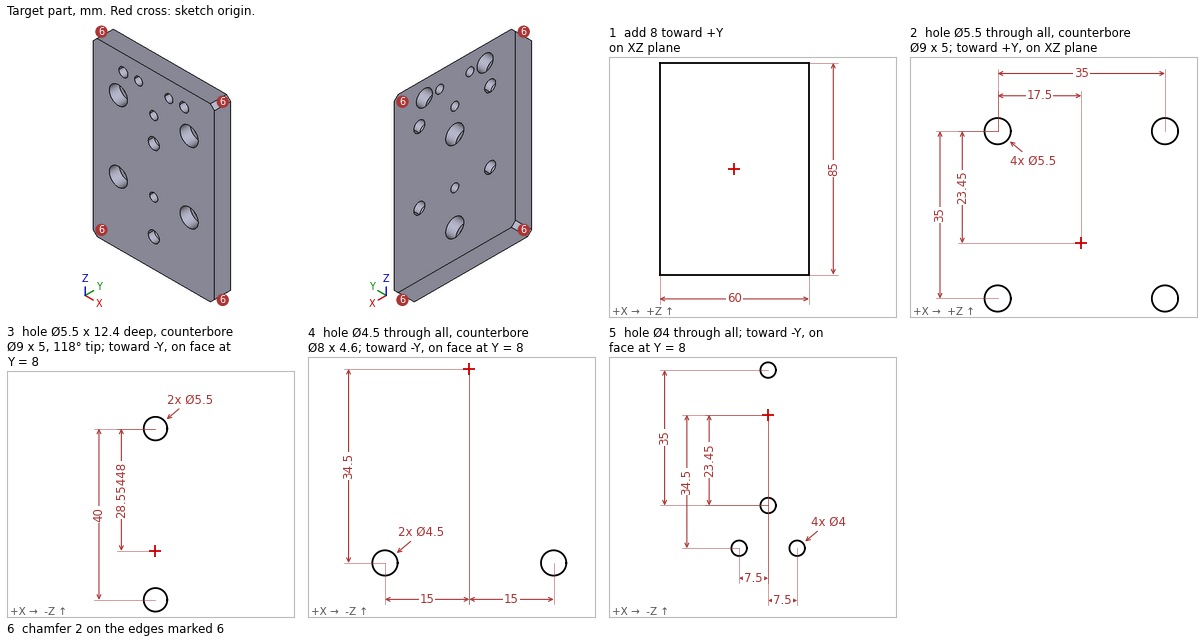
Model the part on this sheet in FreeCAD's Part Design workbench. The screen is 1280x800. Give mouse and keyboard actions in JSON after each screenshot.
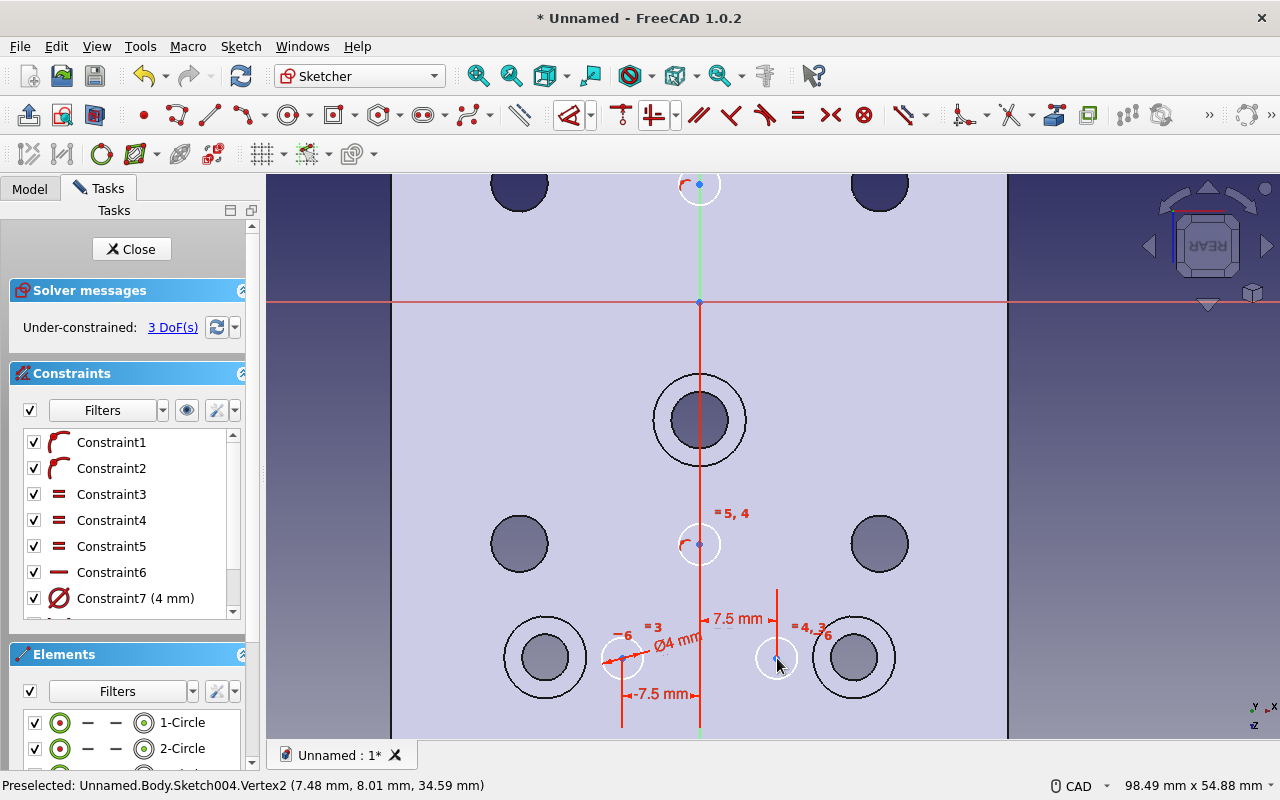
{"action": "left_click", "coordinate": [700, 545]}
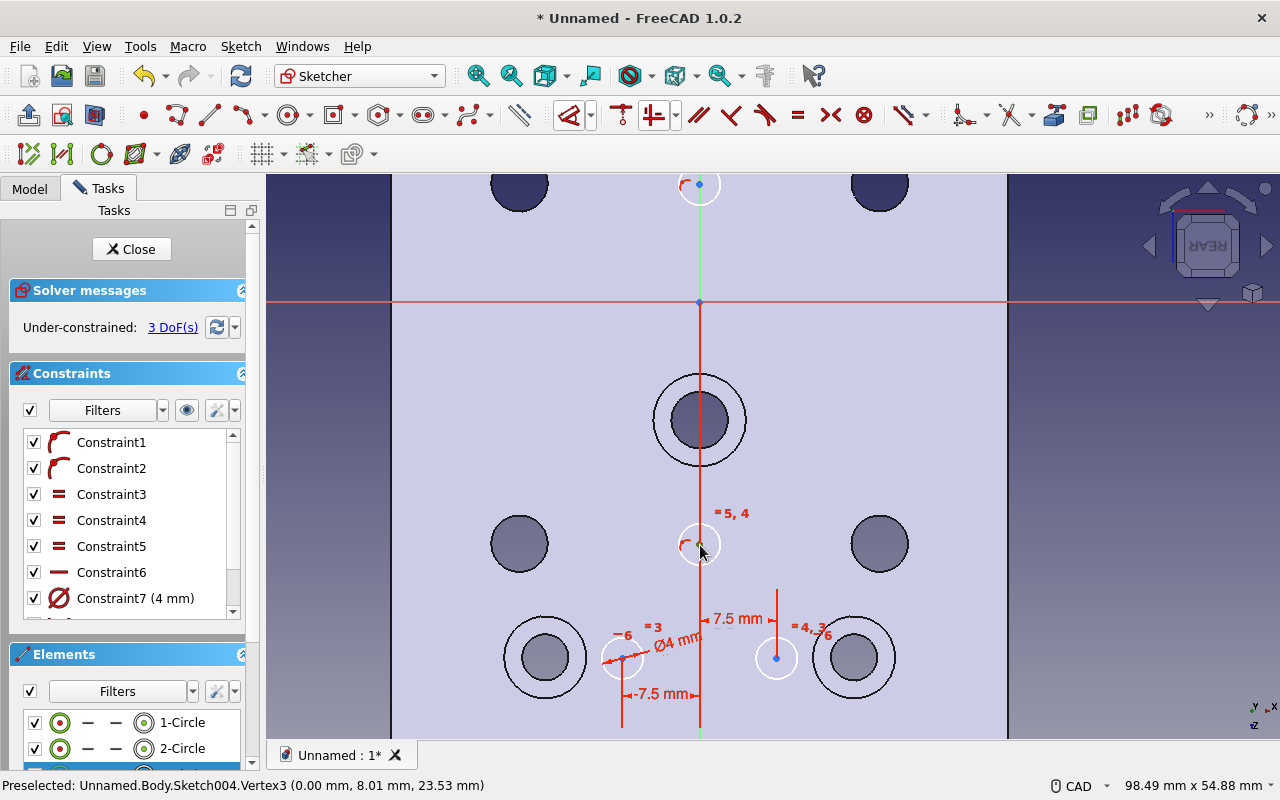
{"action": "scroll", "coordinate": [714, 530], "scroll_direction": "down", "scroll_amount": 2}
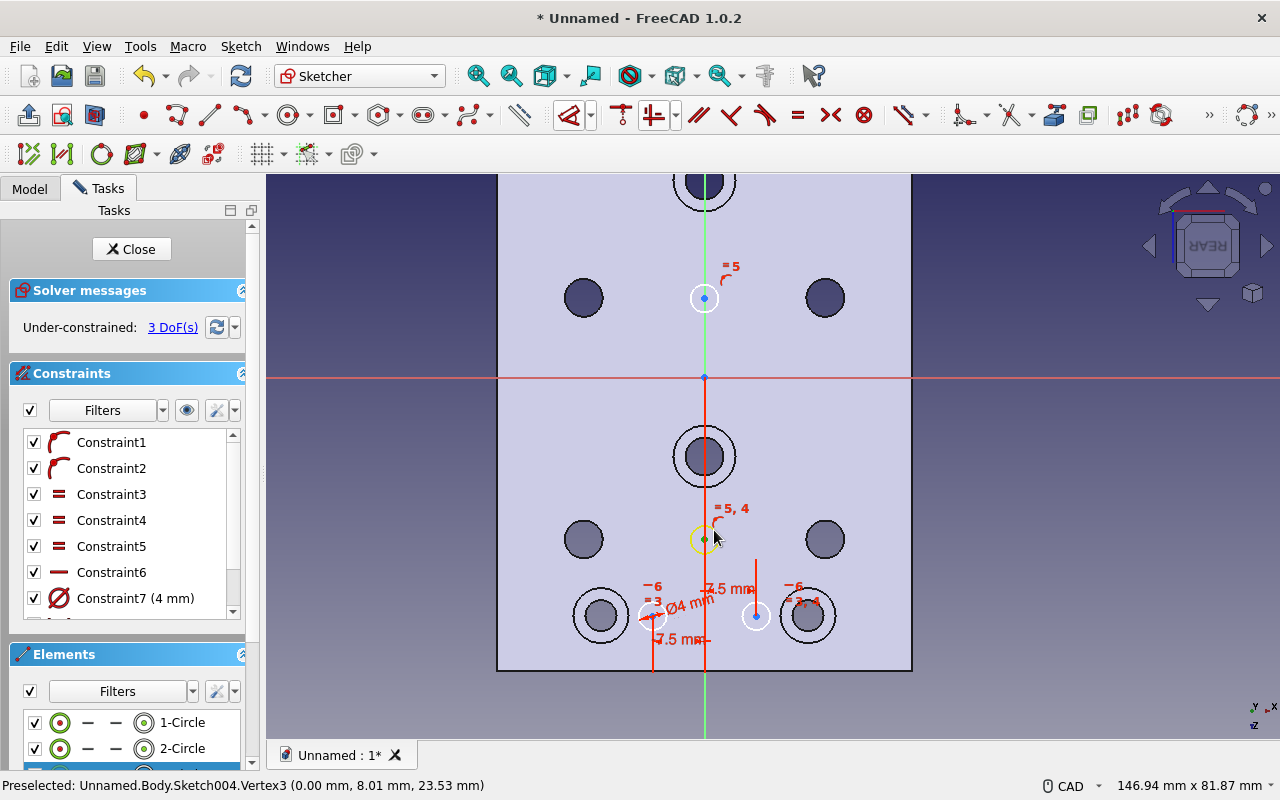
{"action": "left_click", "coordinate": [705, 299]}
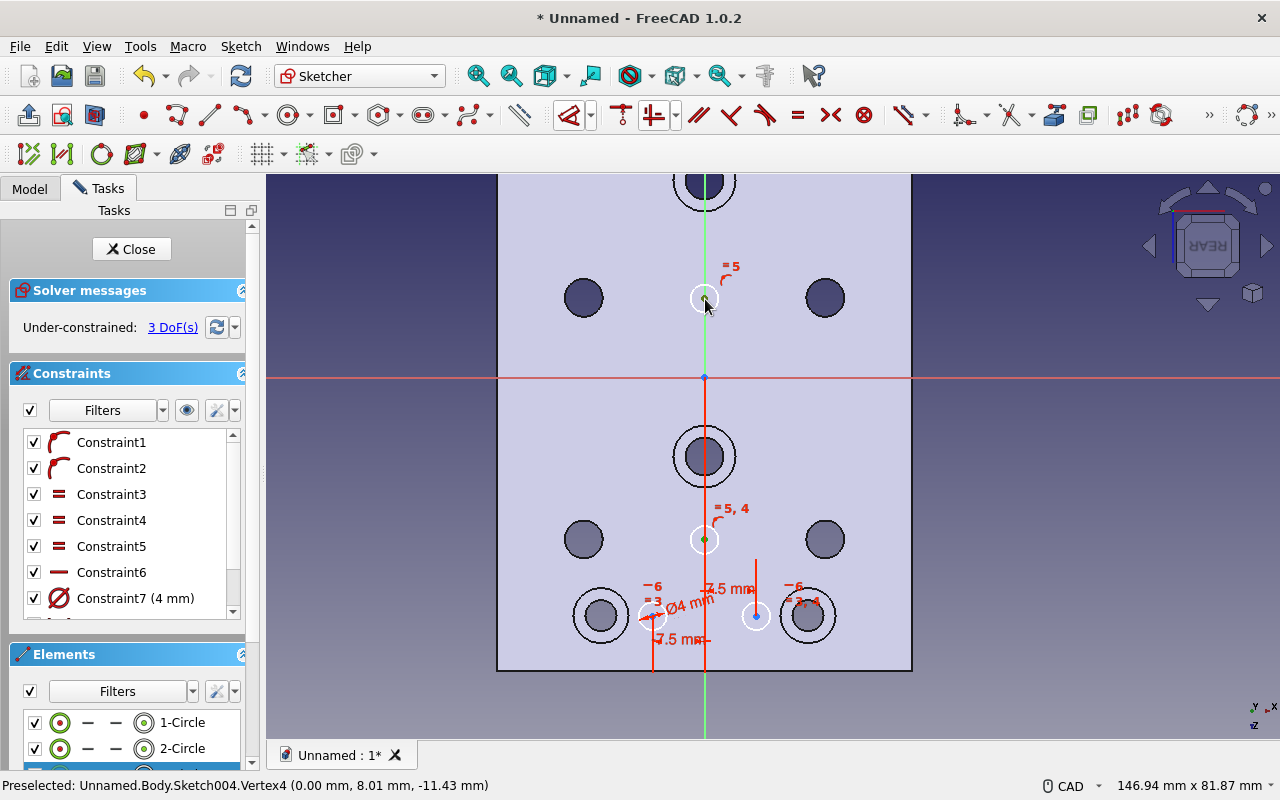
{"action": "key", "text": "i"}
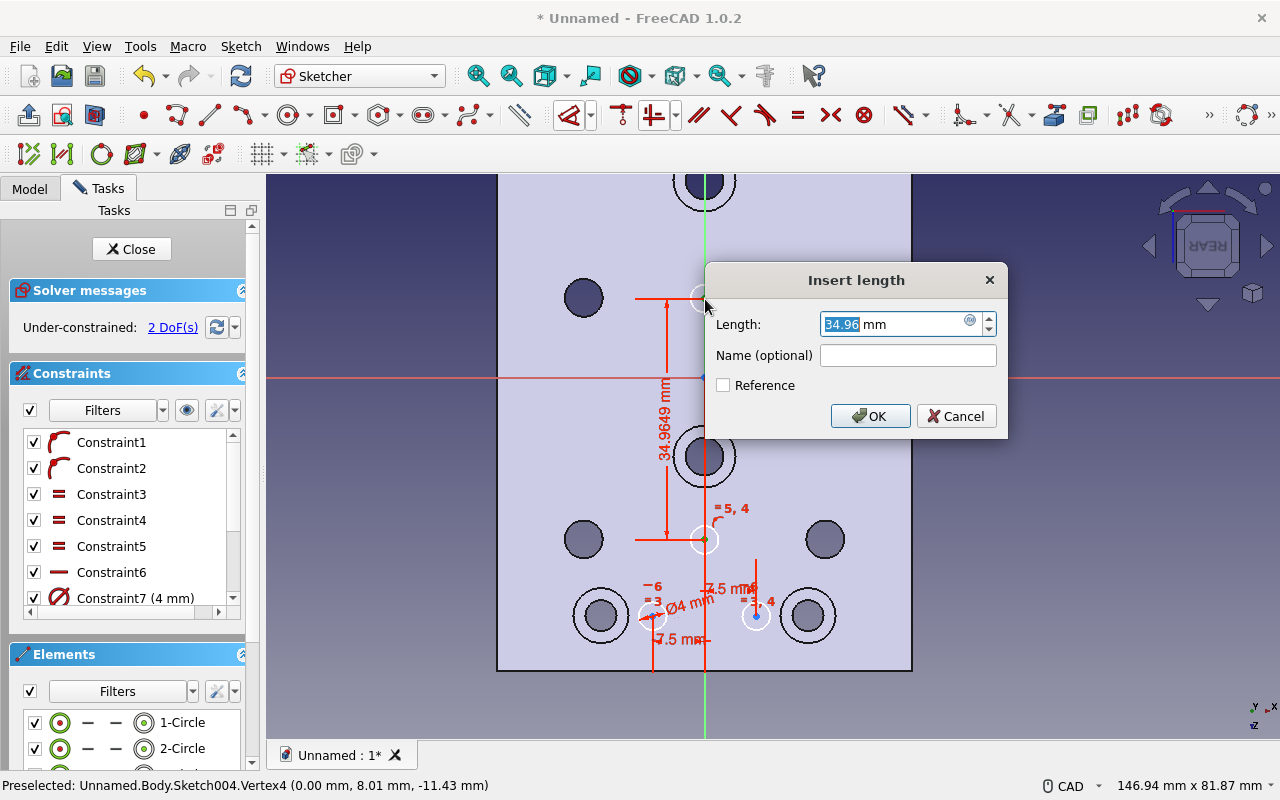
{"action": "type", "text": "35"}
{"action": "key", "text": "Return"}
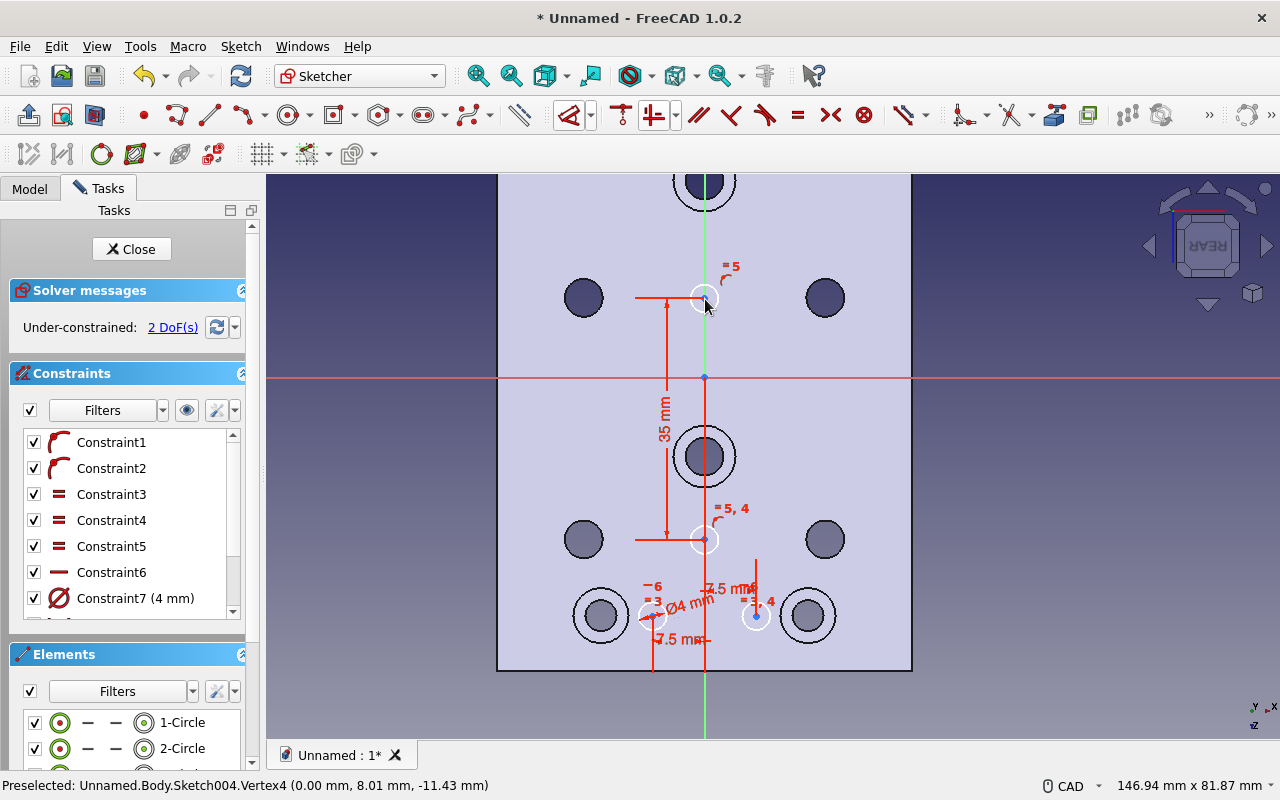
{"action": "left_click", "coordinate": [653, 616]}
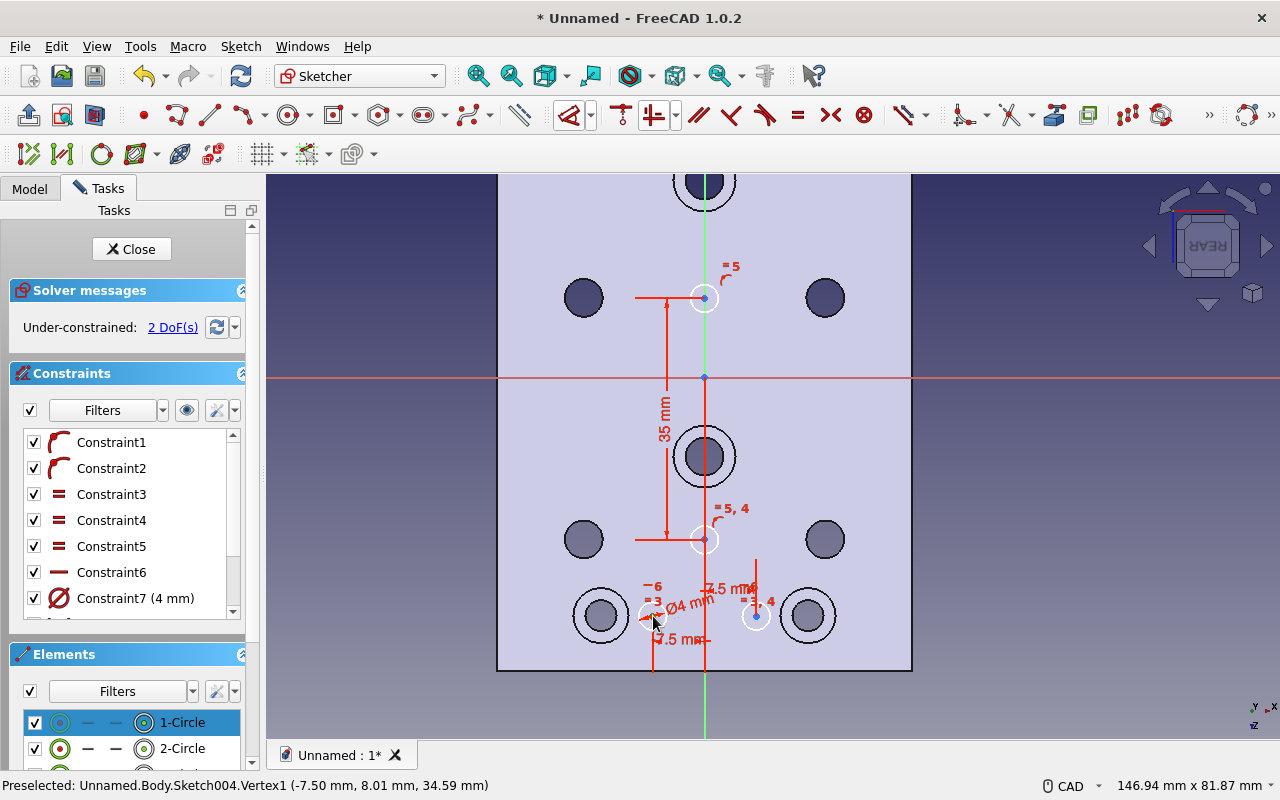
{"action": "key", "text": "i"}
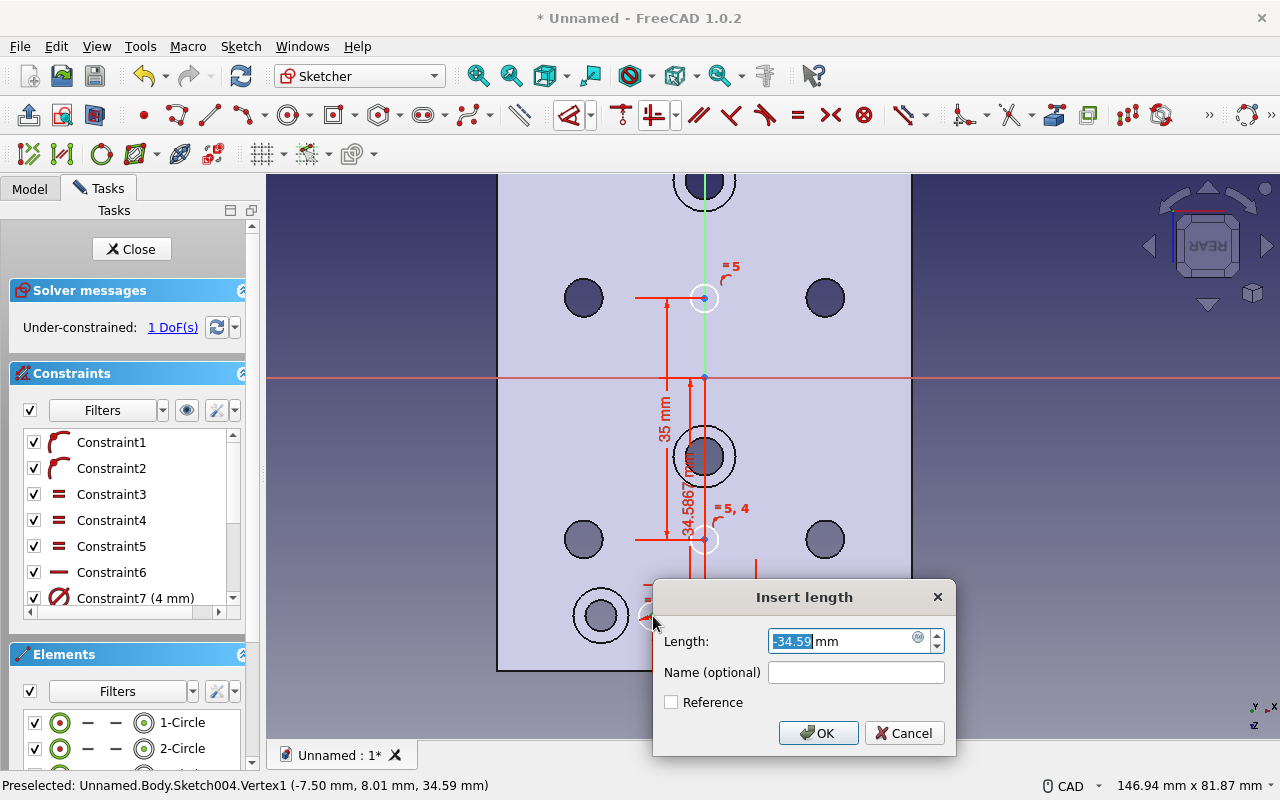
{"action": "type", "text": "-34.5"}
{"action": "key", "text": "Return"}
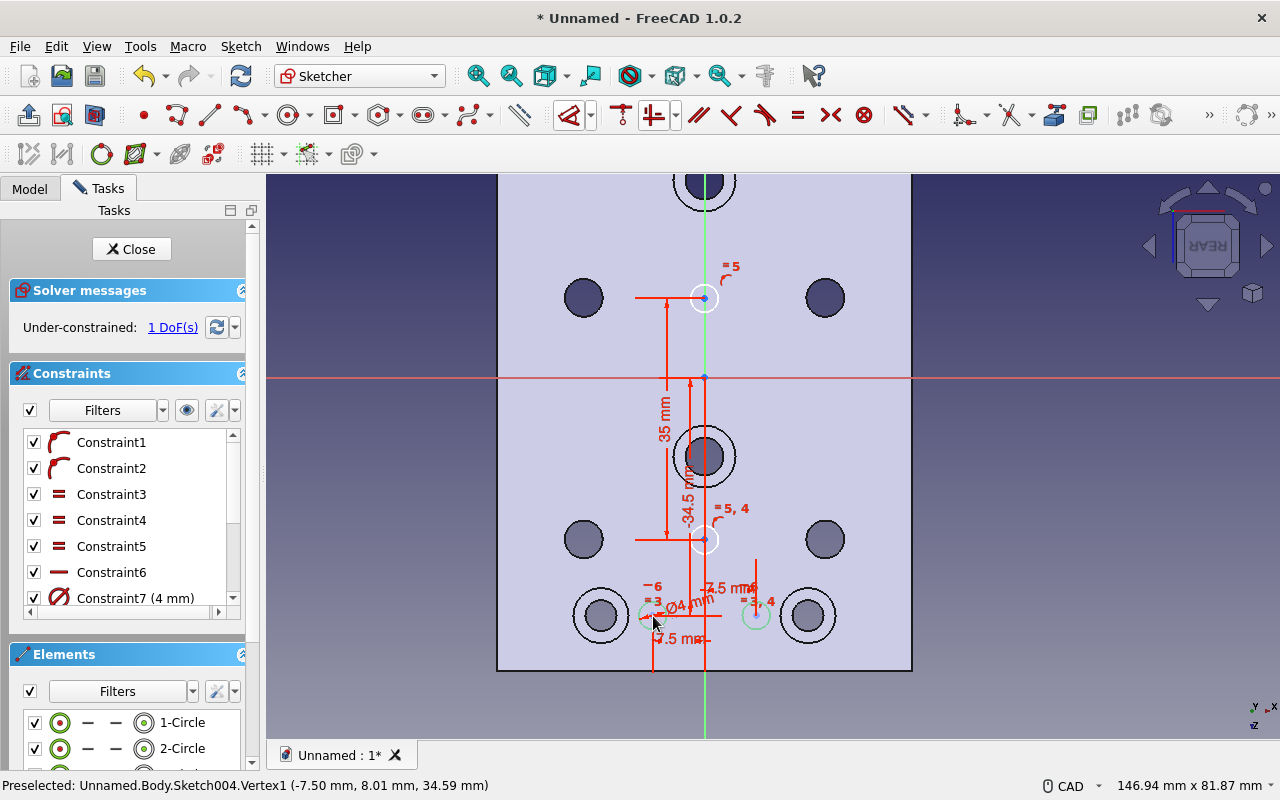
{"action": "left_click", "coordinate": [705, 540]}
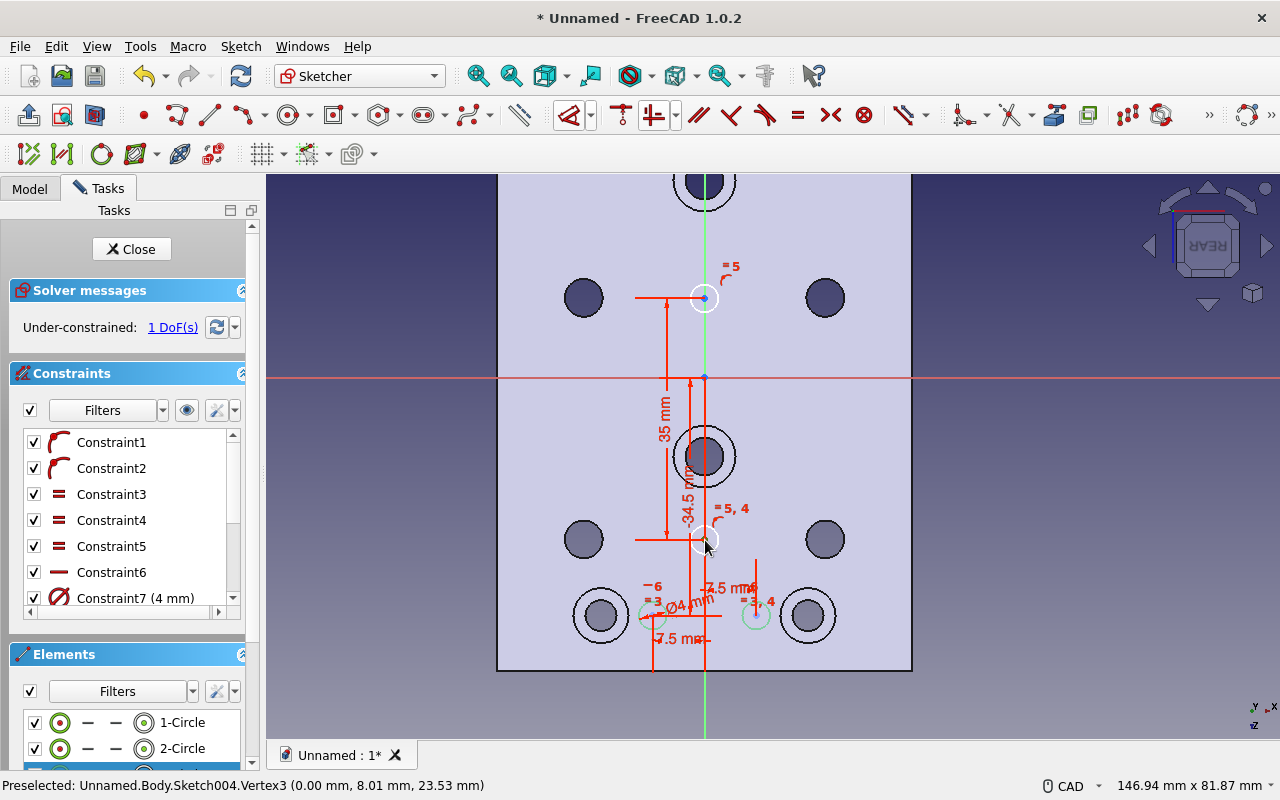
{"action": "key", "text": "i"}